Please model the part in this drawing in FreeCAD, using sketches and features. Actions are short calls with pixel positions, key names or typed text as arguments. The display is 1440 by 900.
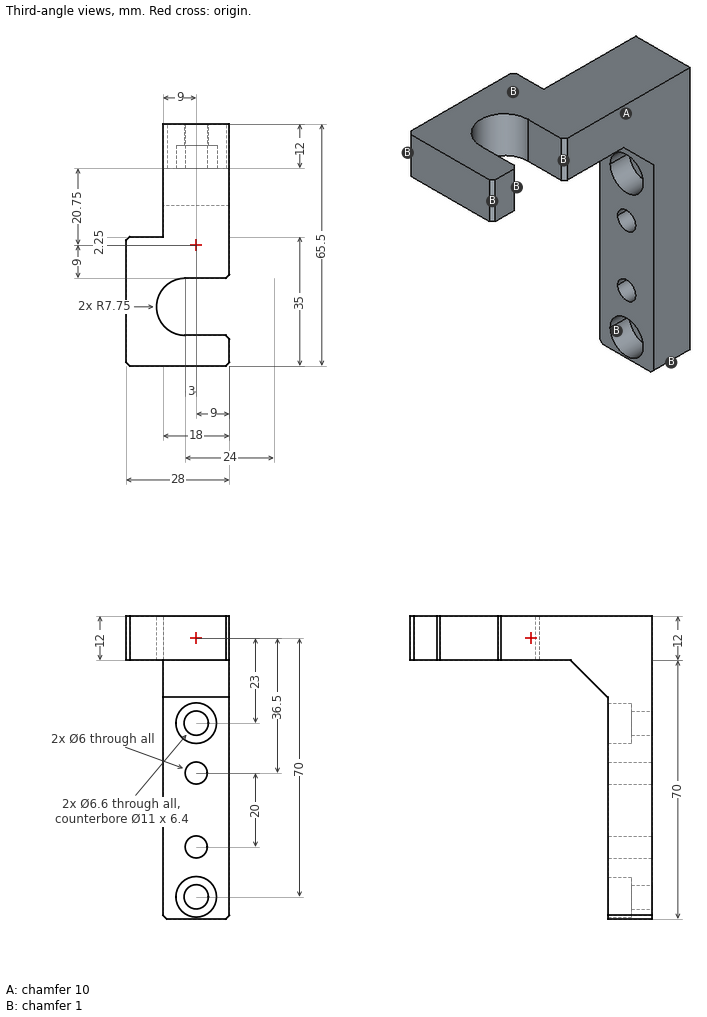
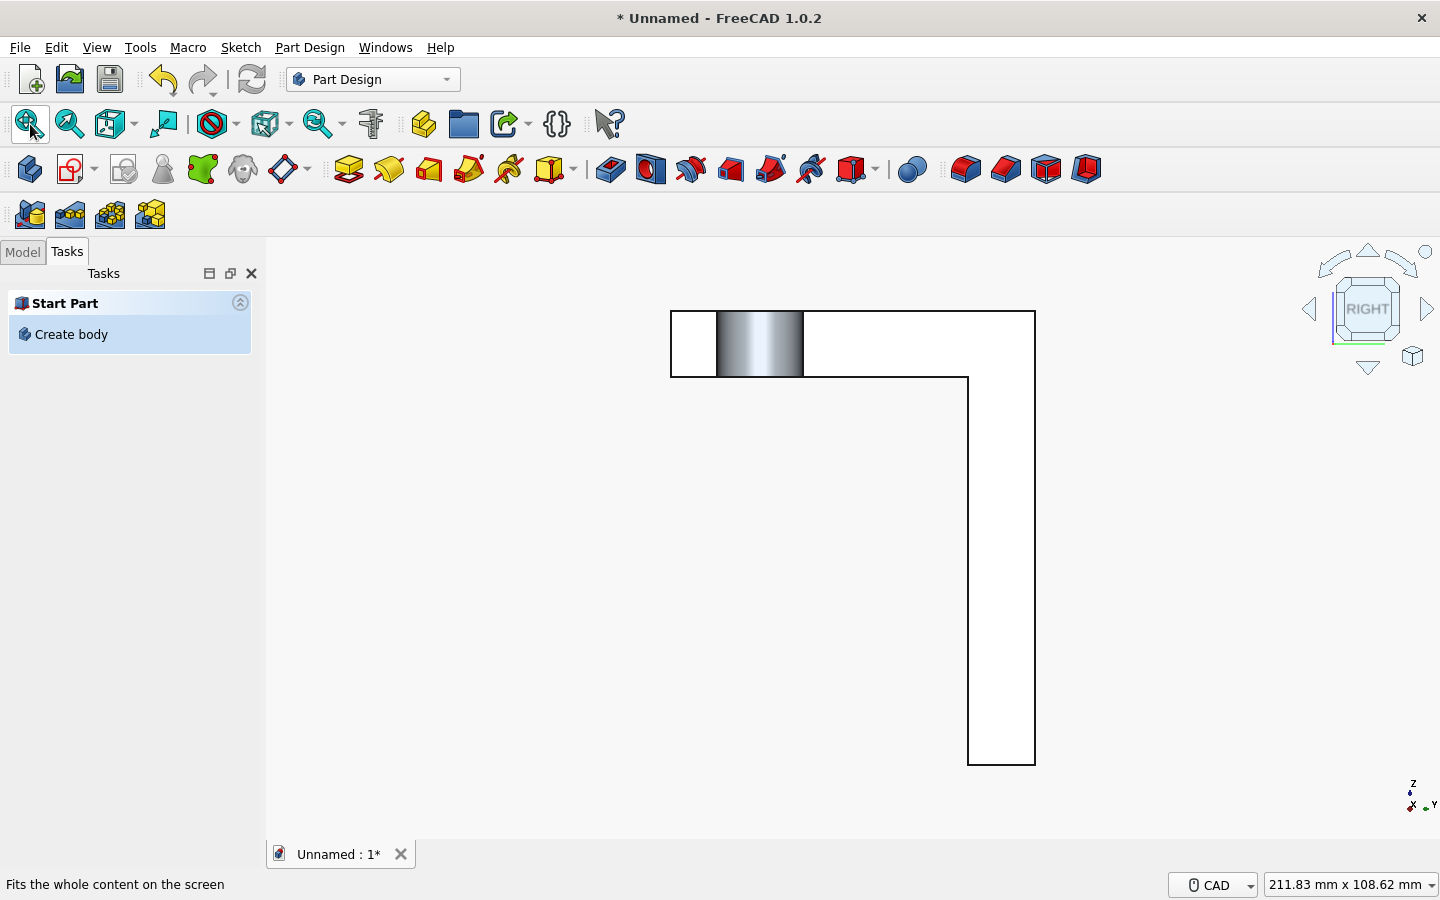
key(5)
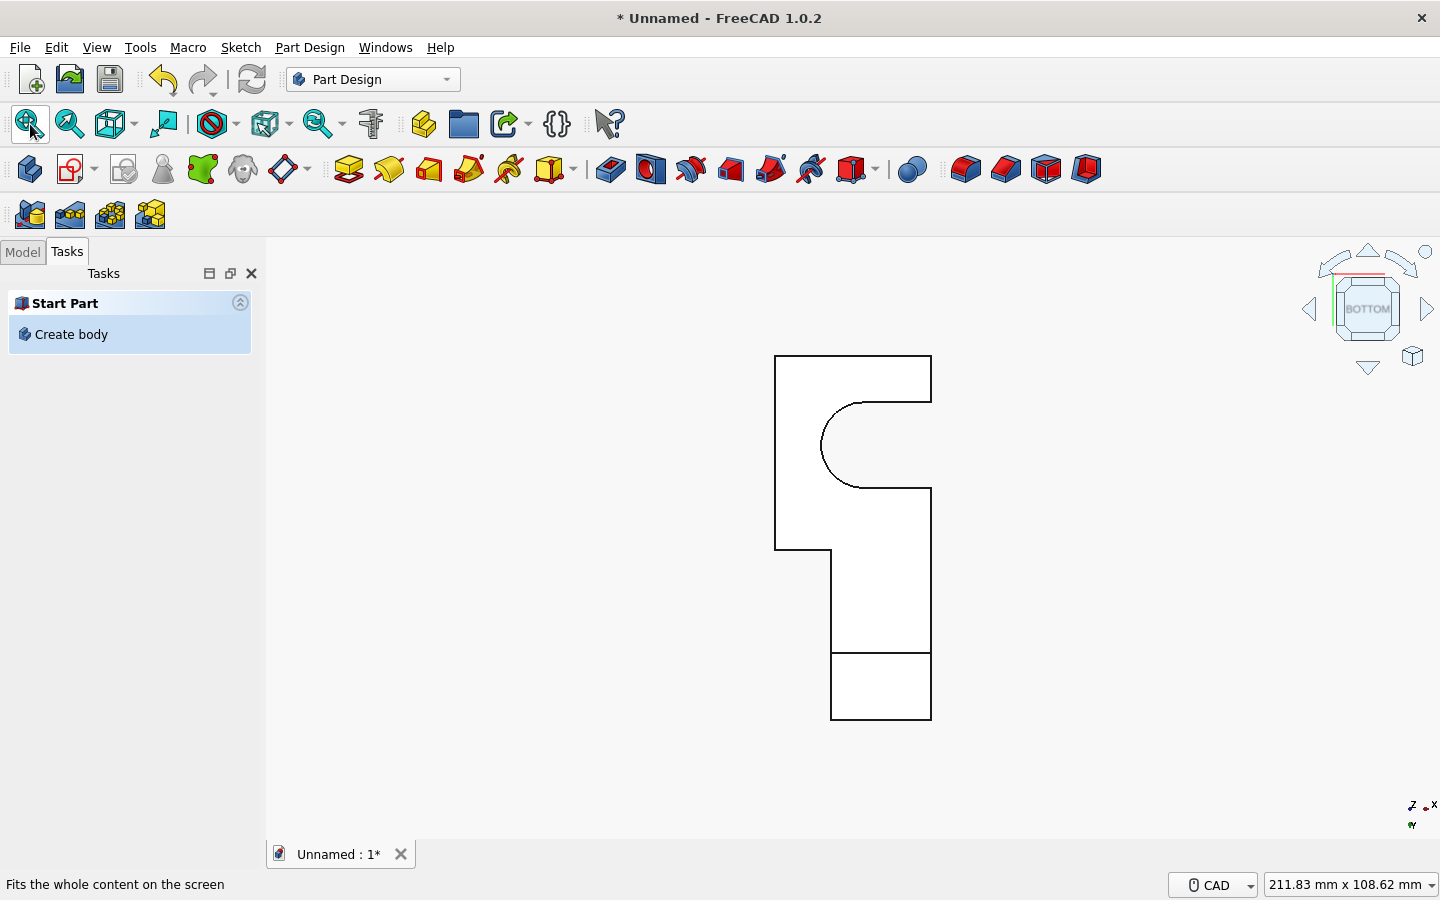
key(4)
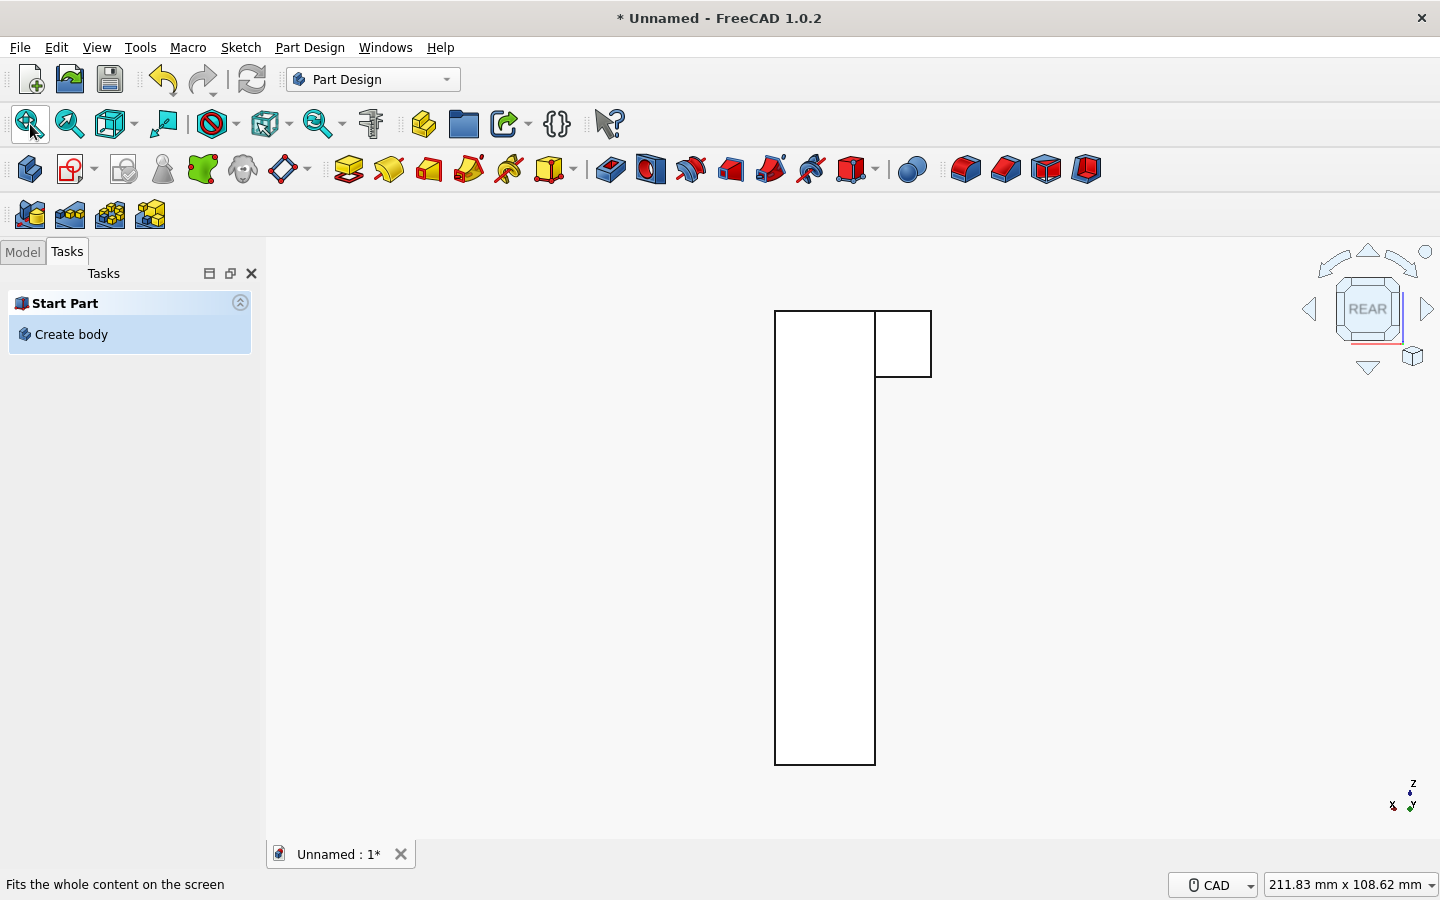
key(6)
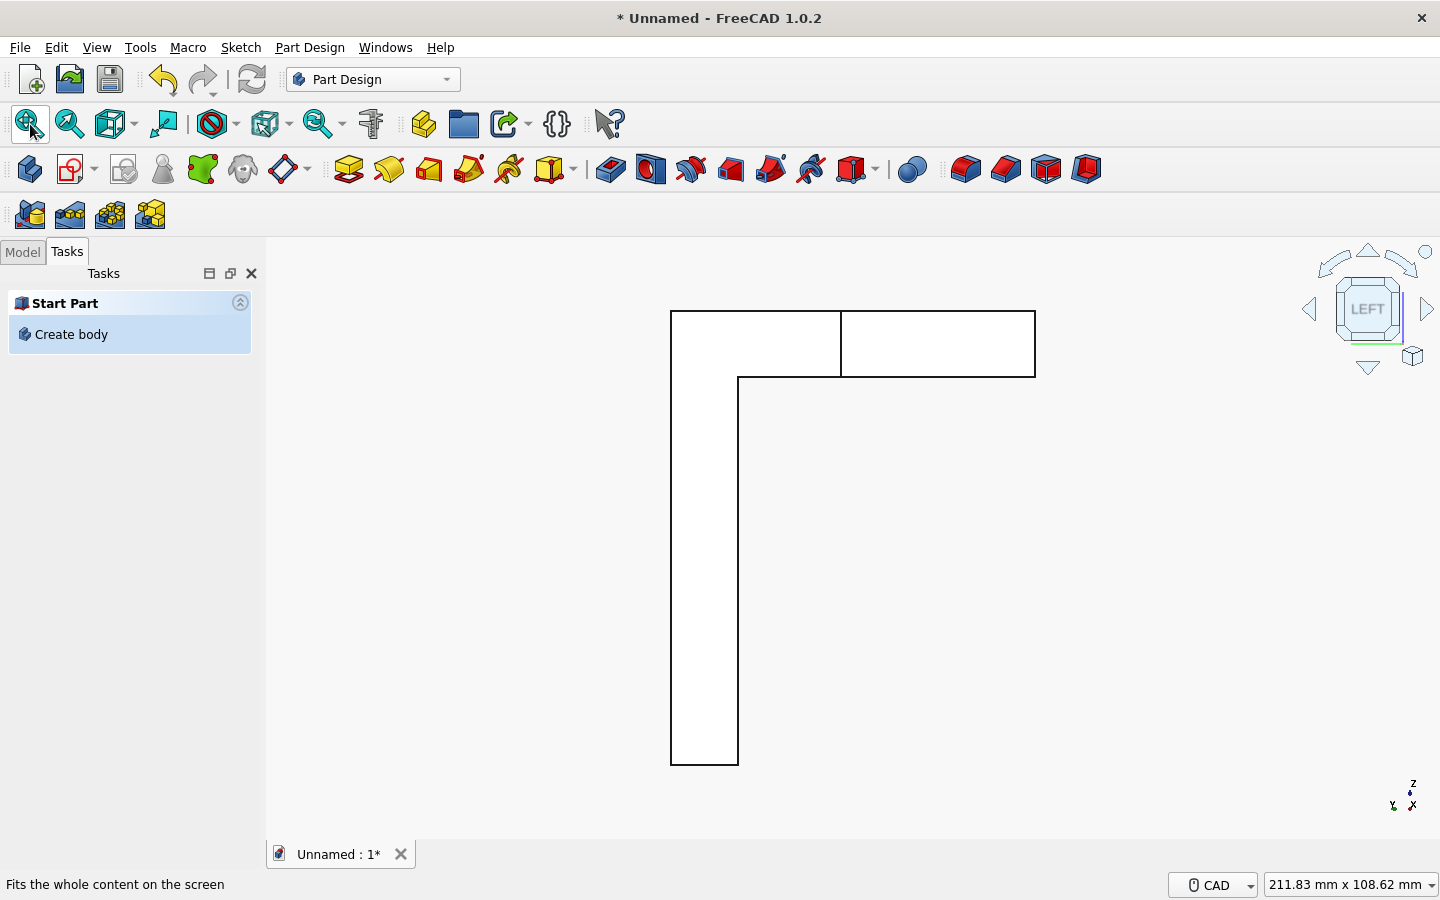
key(v)
key(3)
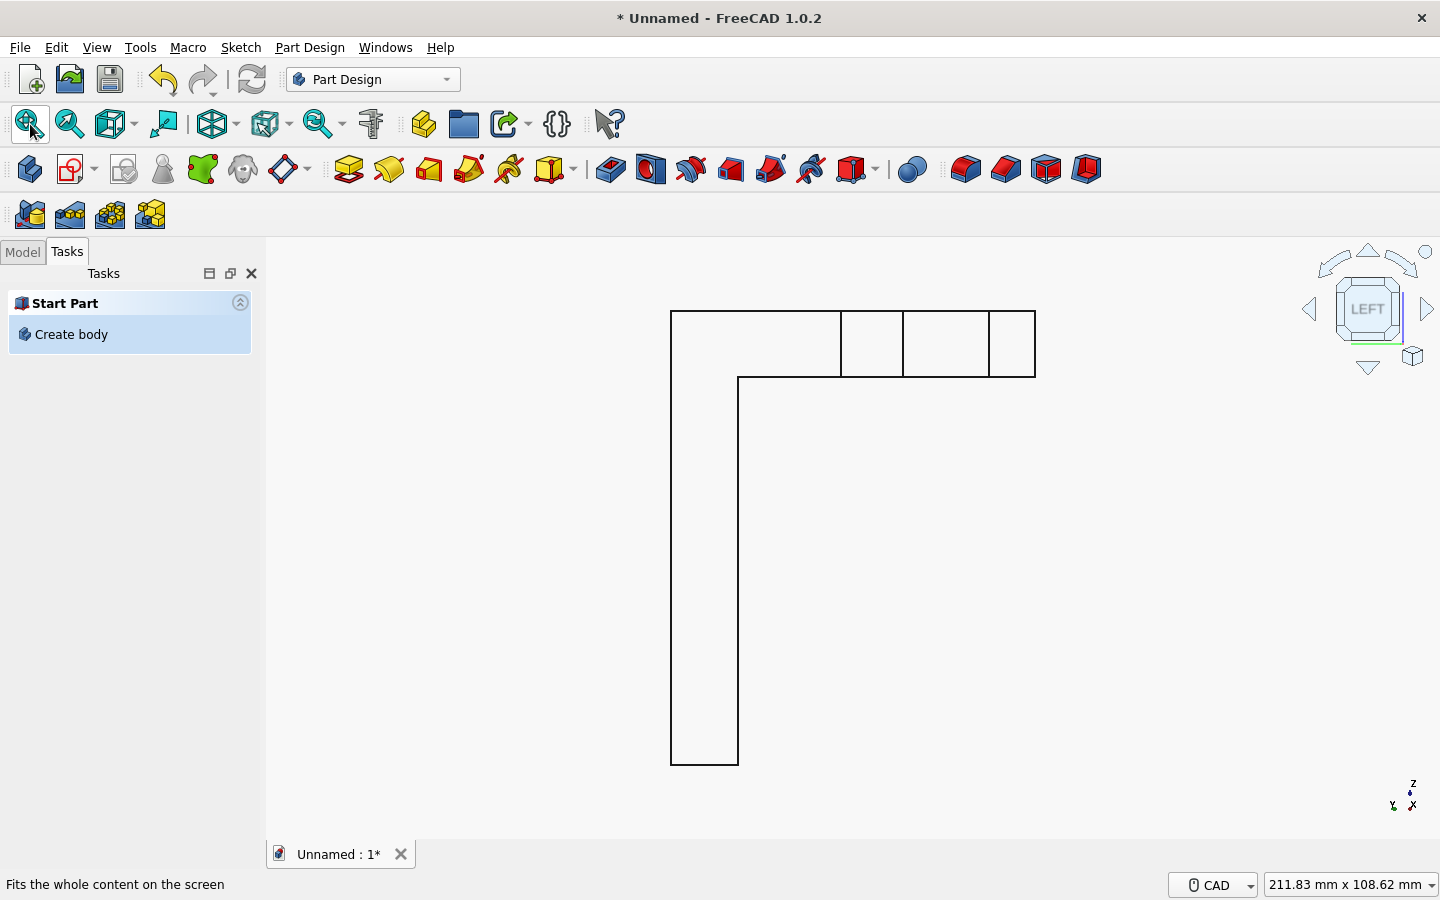
key(0)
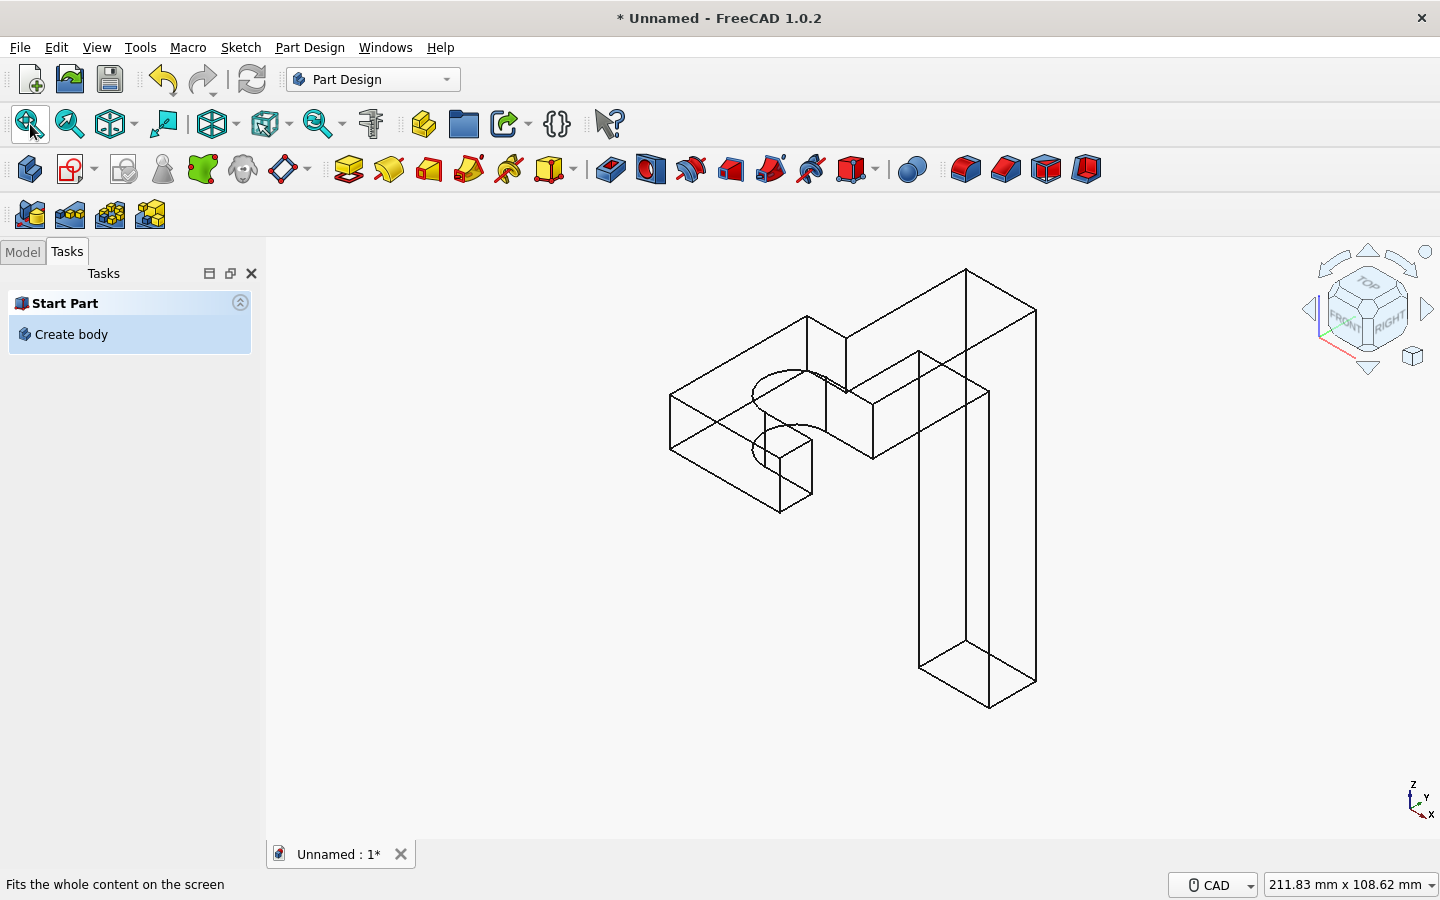
click(954, 370)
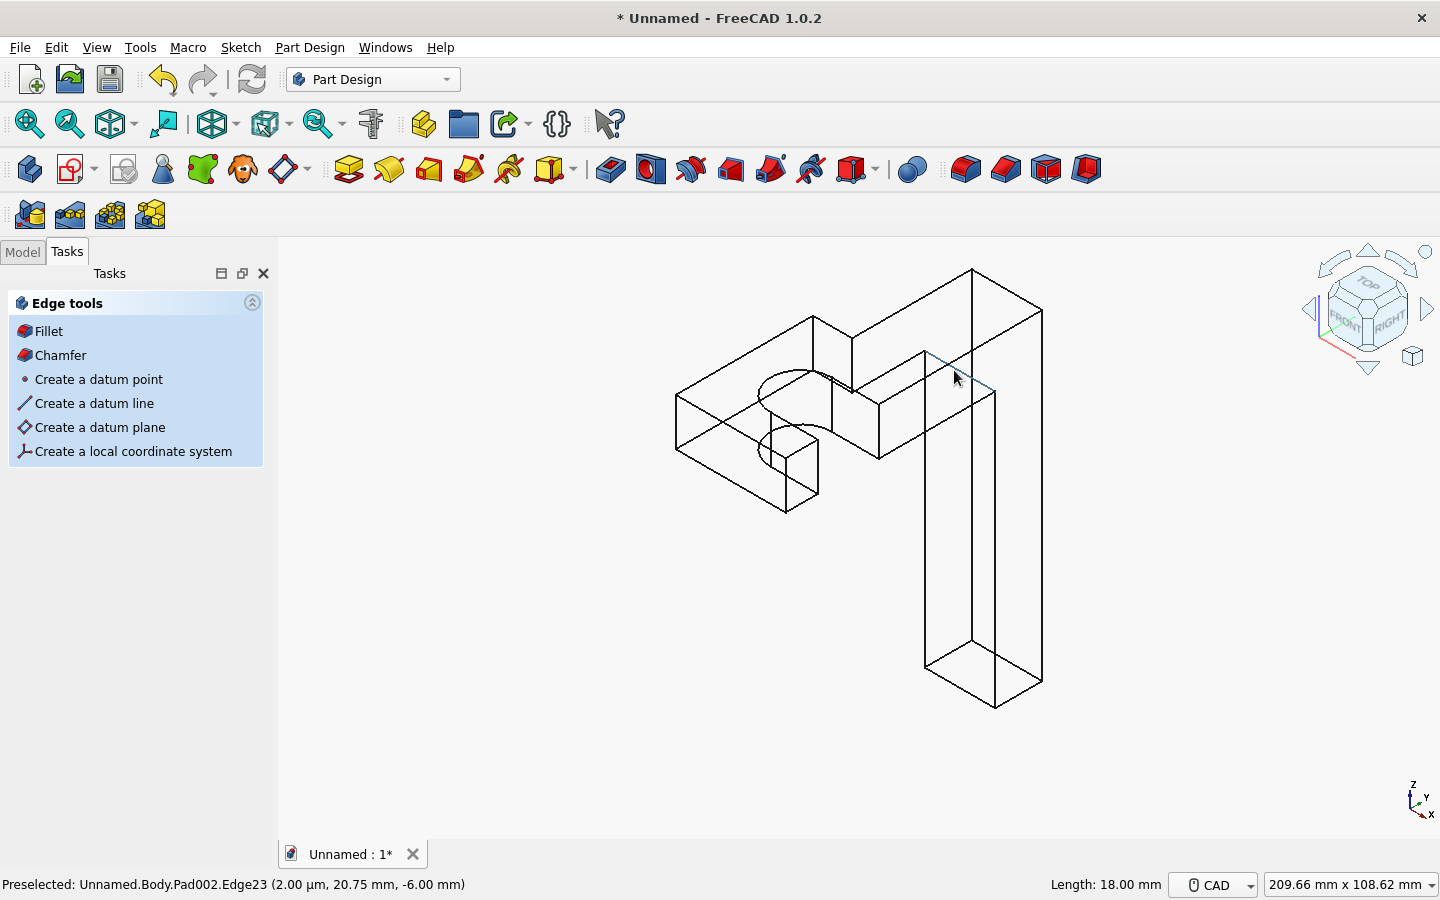
key(v)
key(1)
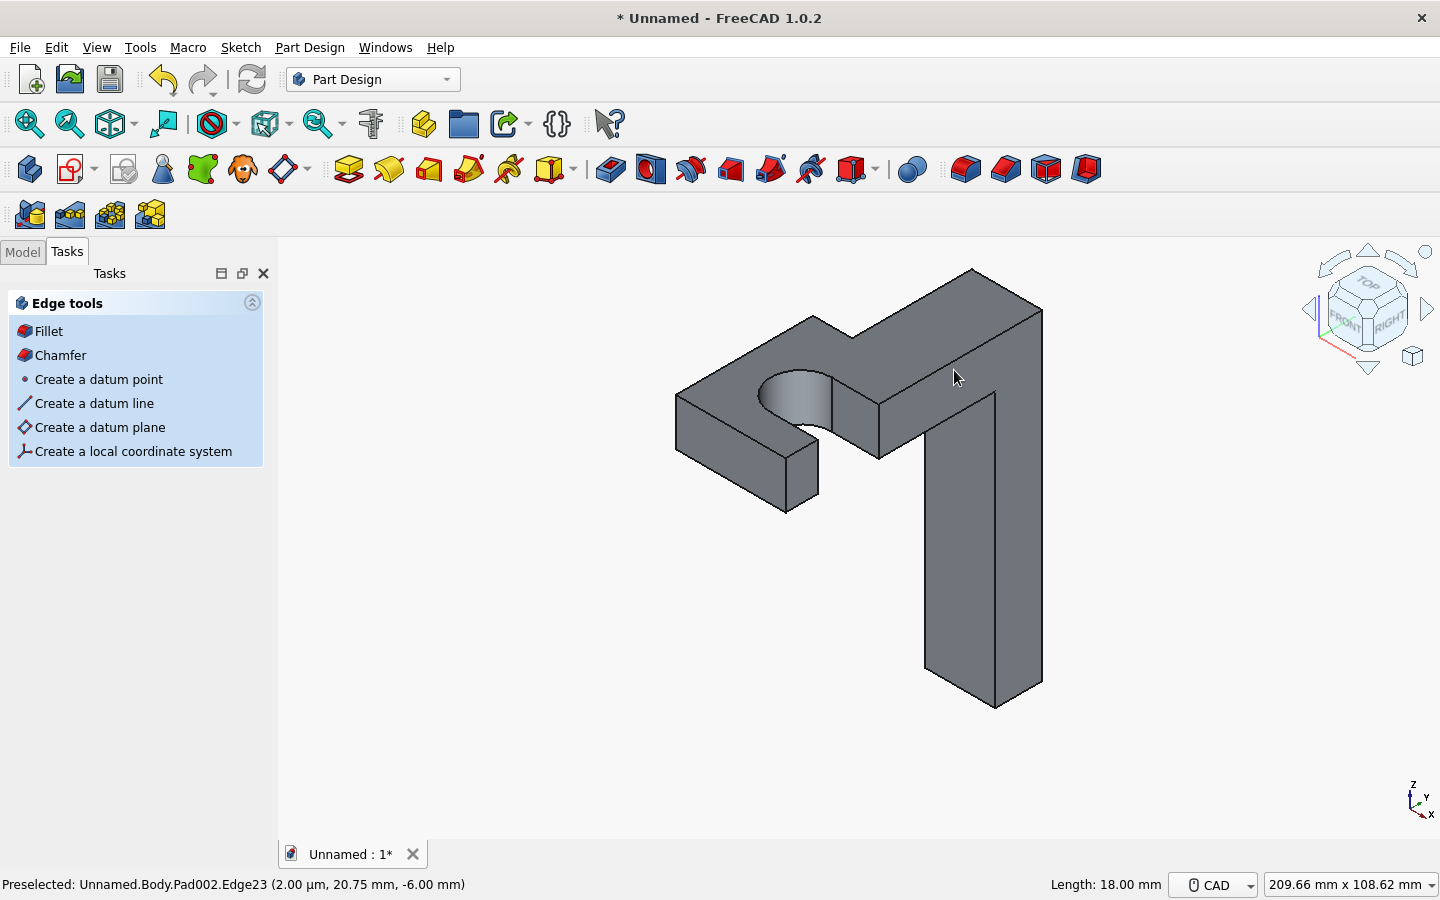
click(1006, 170)